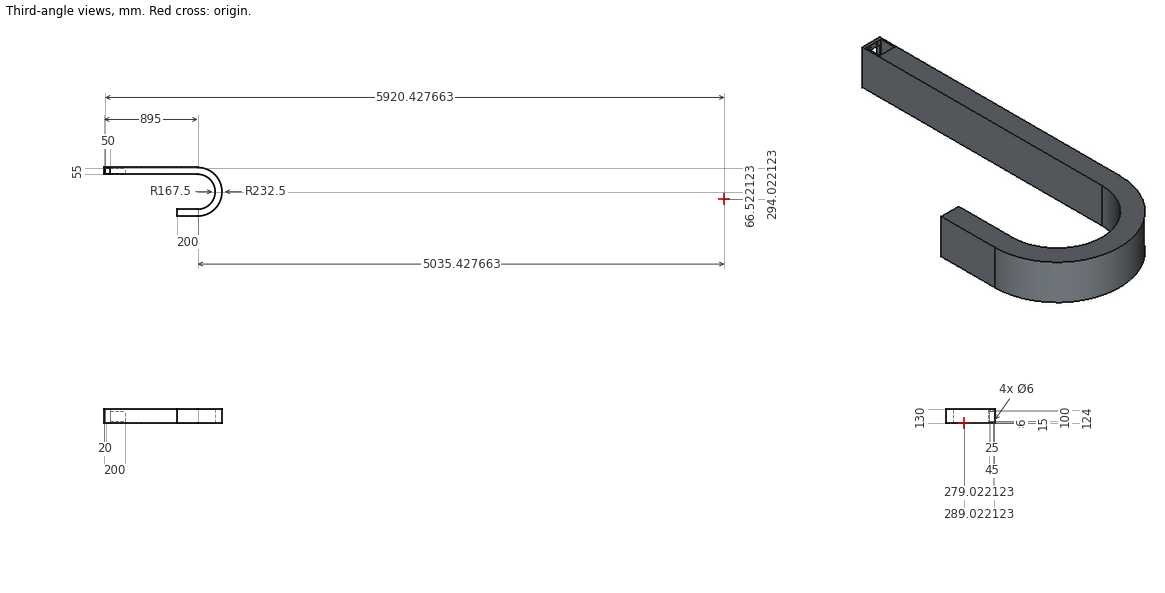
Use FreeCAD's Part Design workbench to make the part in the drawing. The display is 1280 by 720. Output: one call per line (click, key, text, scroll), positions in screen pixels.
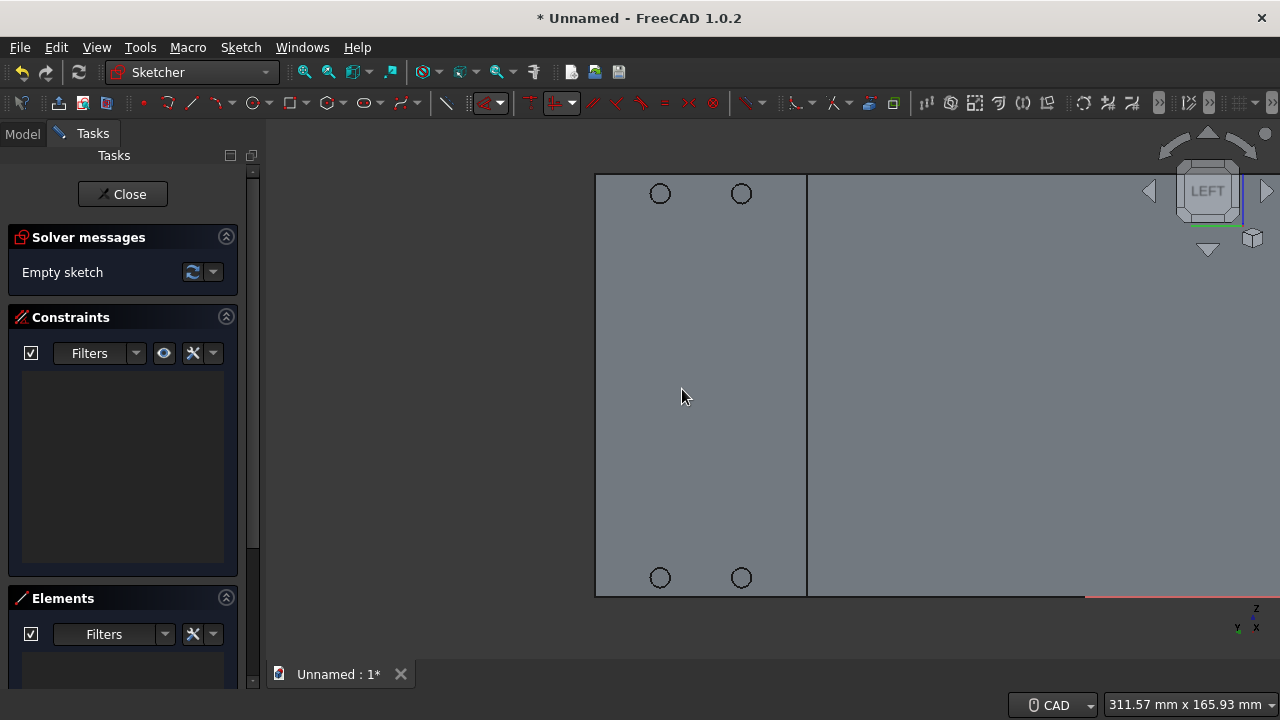
click(290, 104)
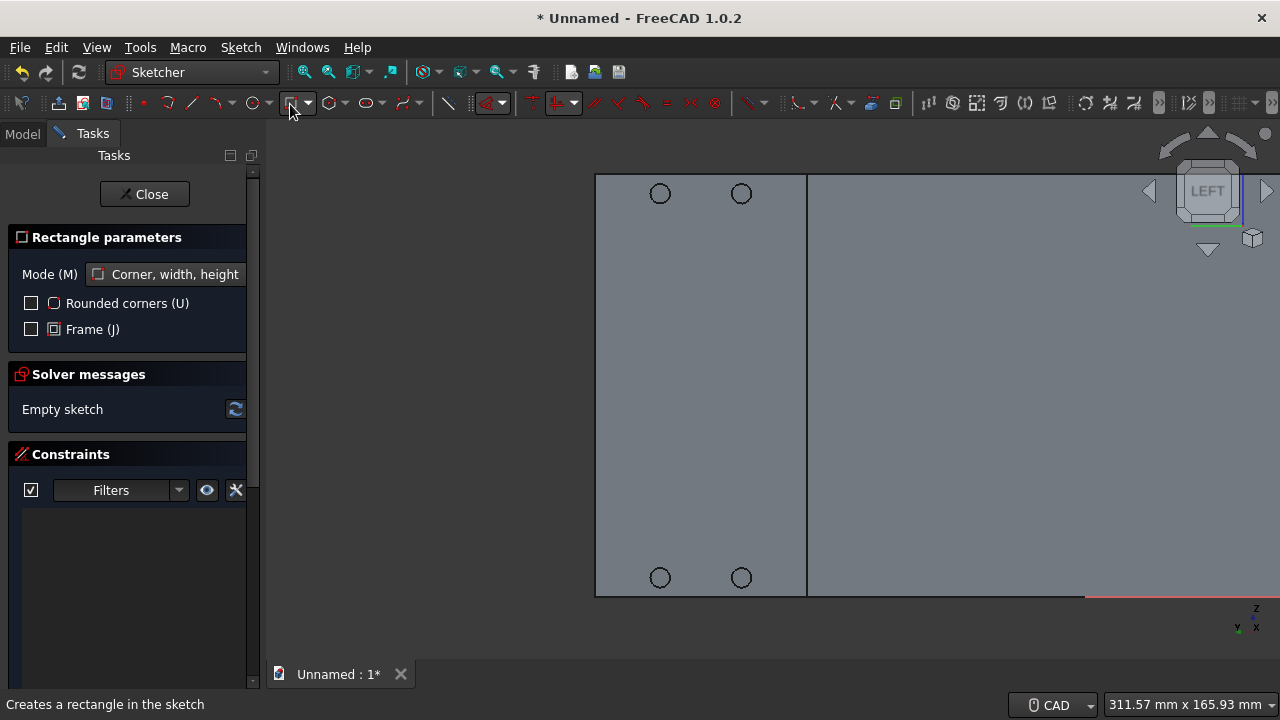
click(628, 223)
move(774, 549)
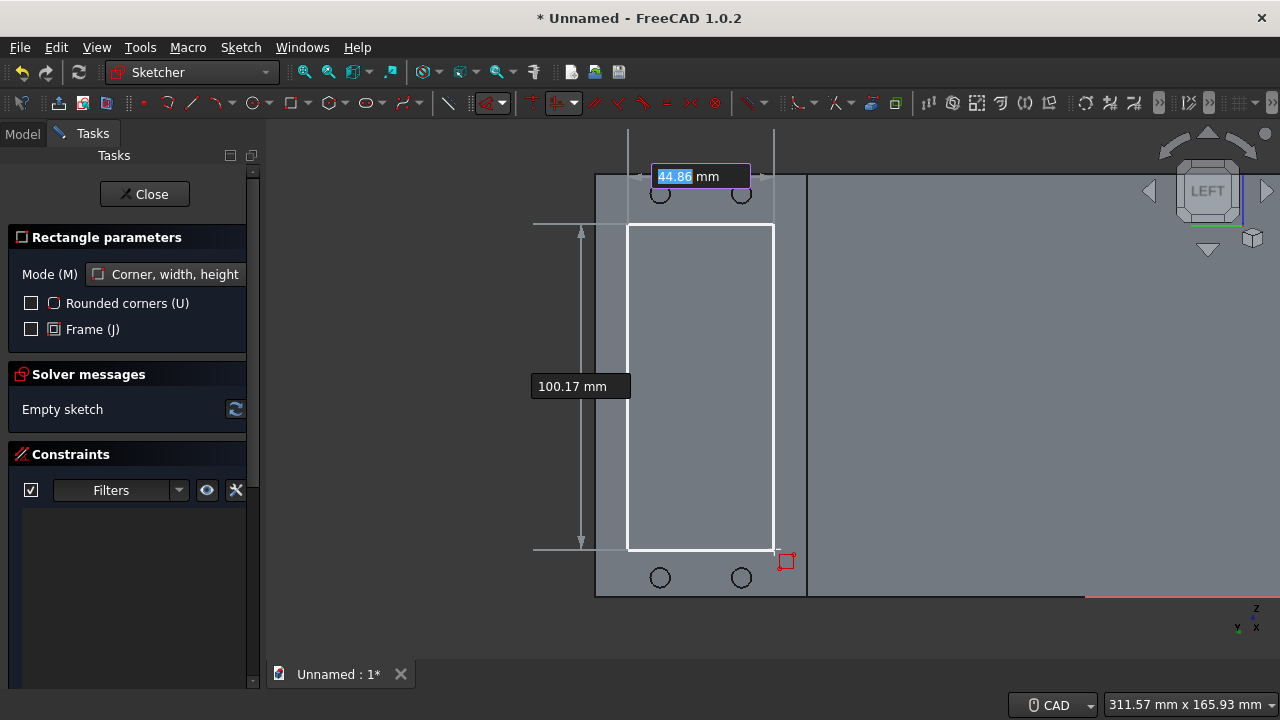
text(45)
key(Tab)
text(100)
key(Return)
key(Escape)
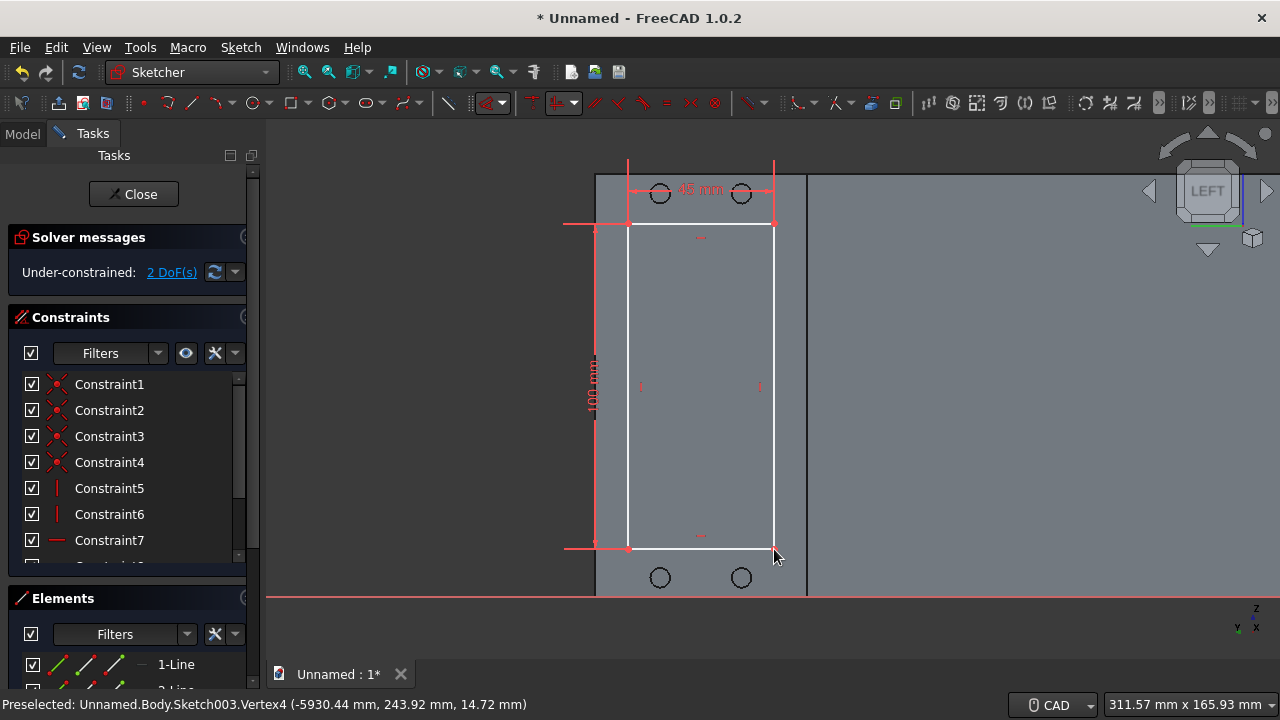
click(628, 549)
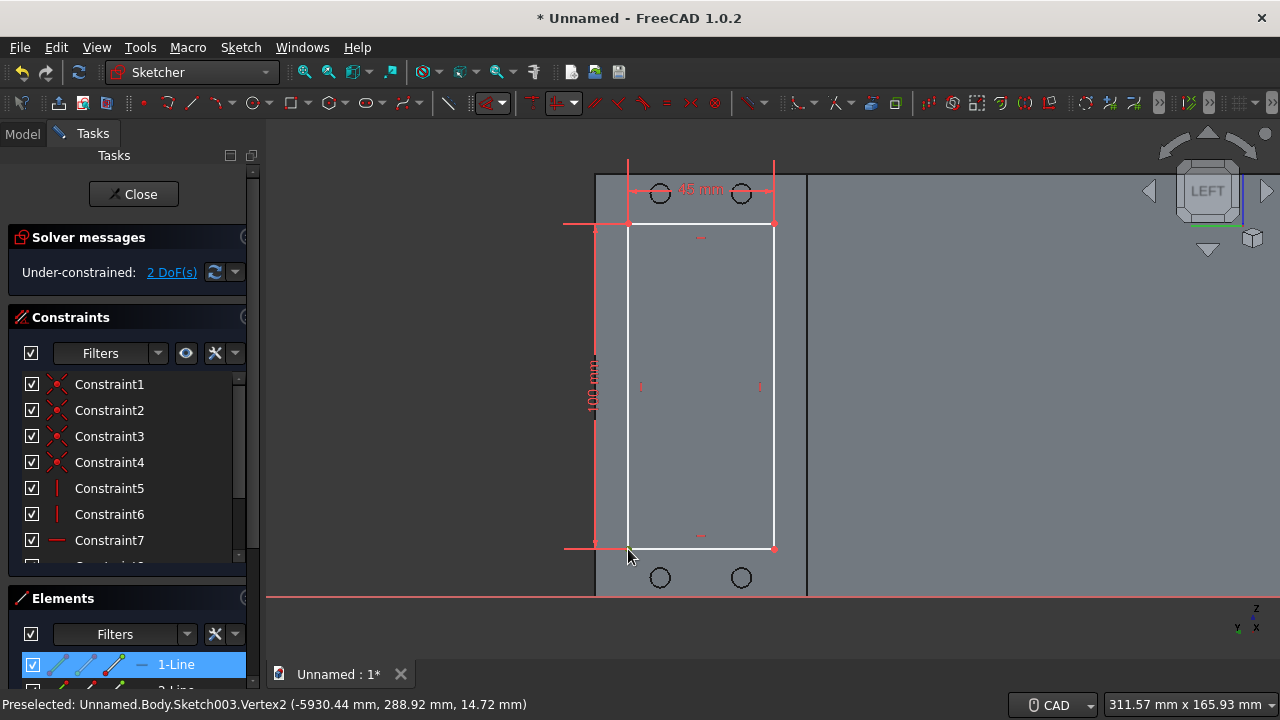
key(i)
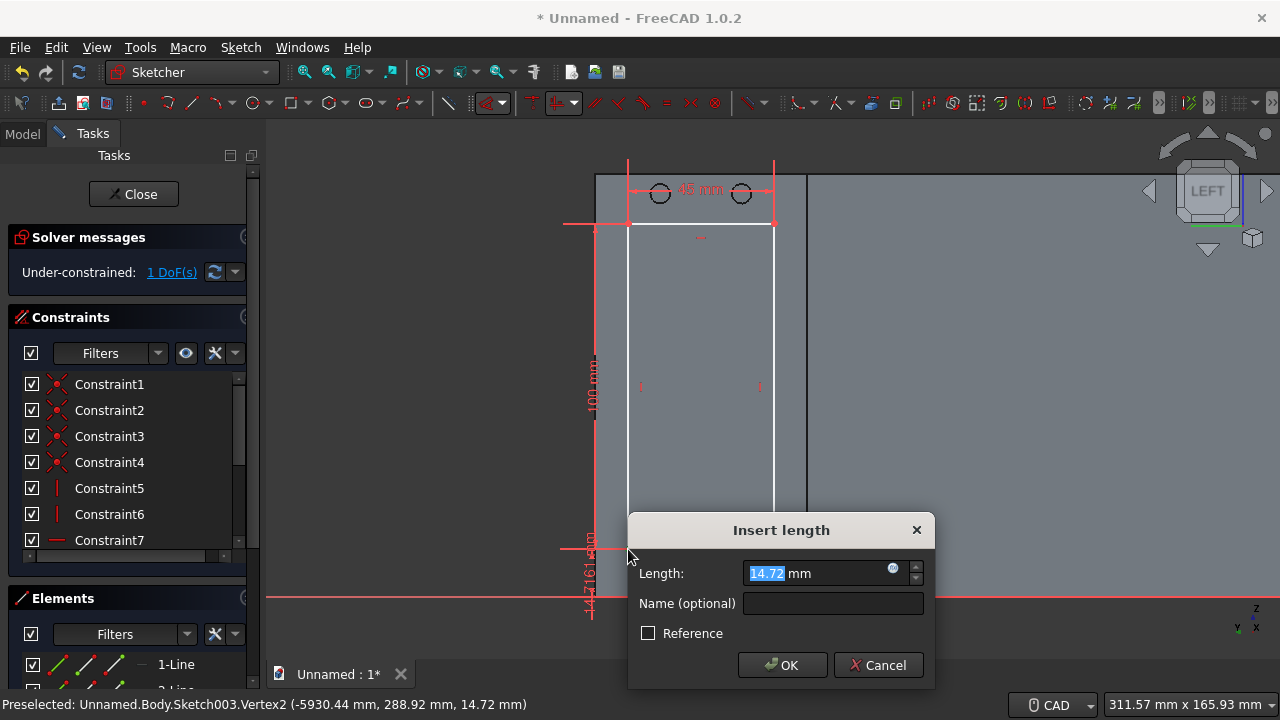
text(15)
key(Return)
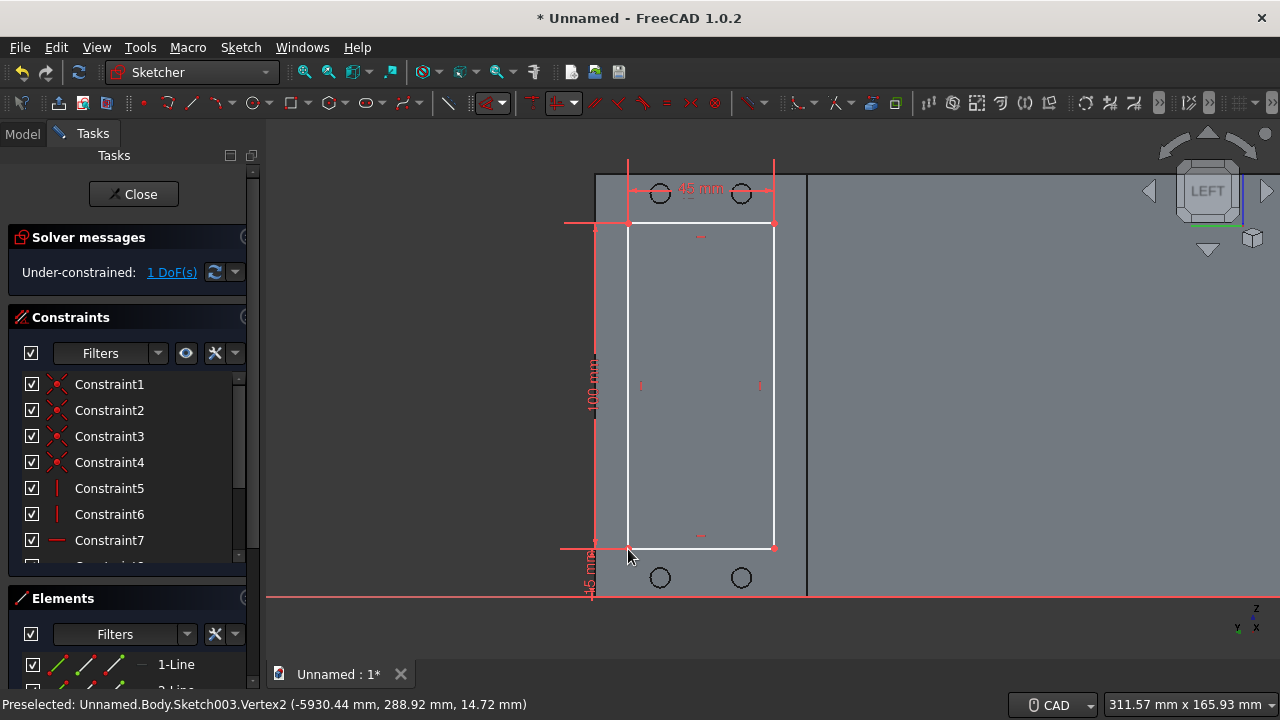
click(628, 223)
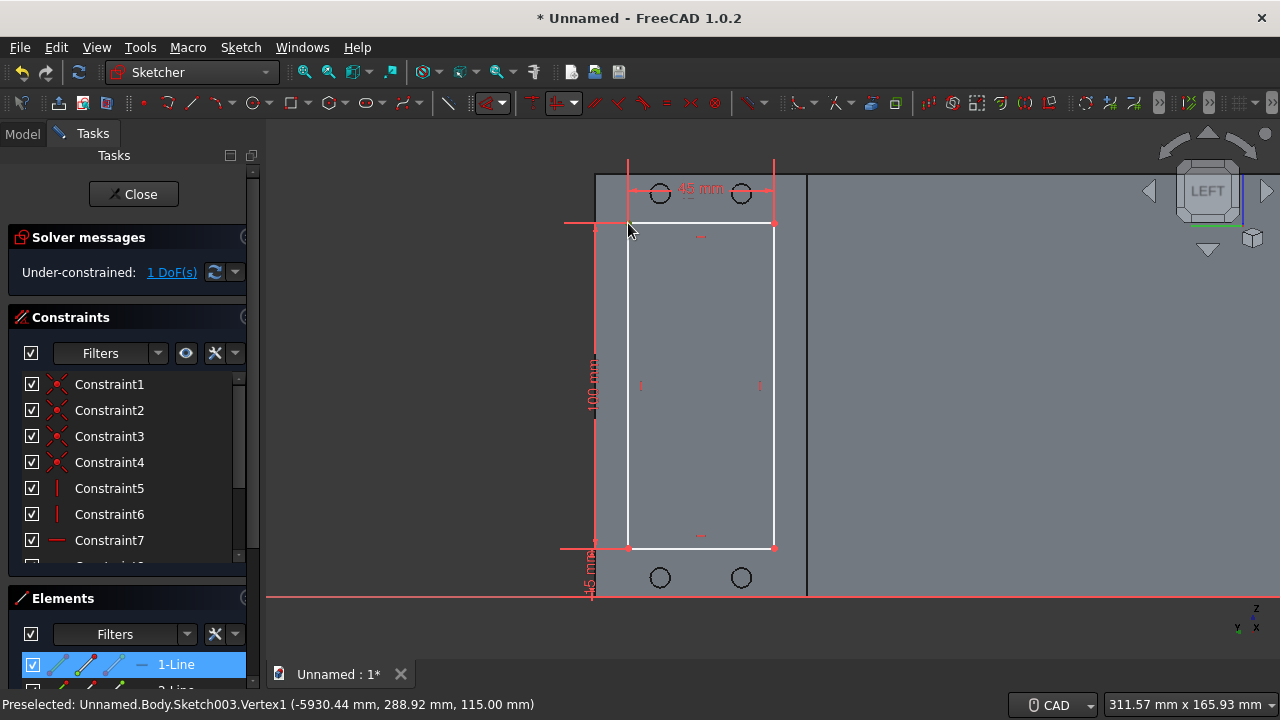
key(l)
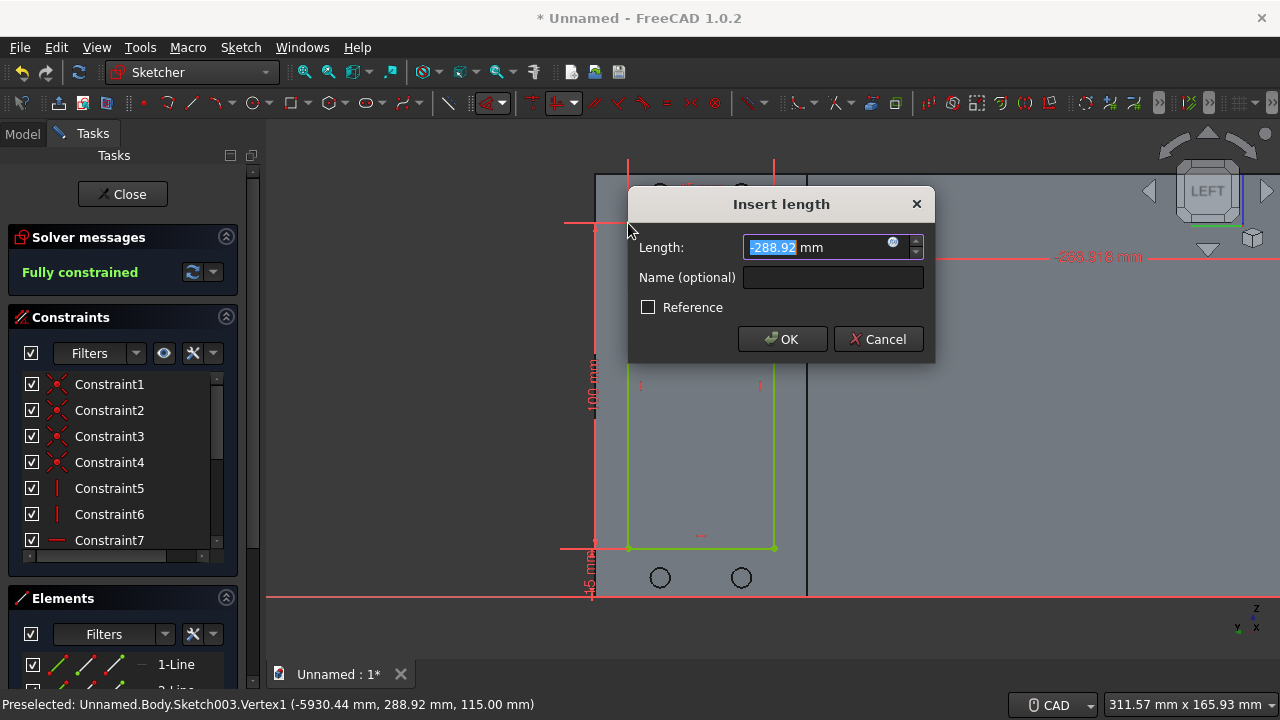
text(-289.022123)
key(Return)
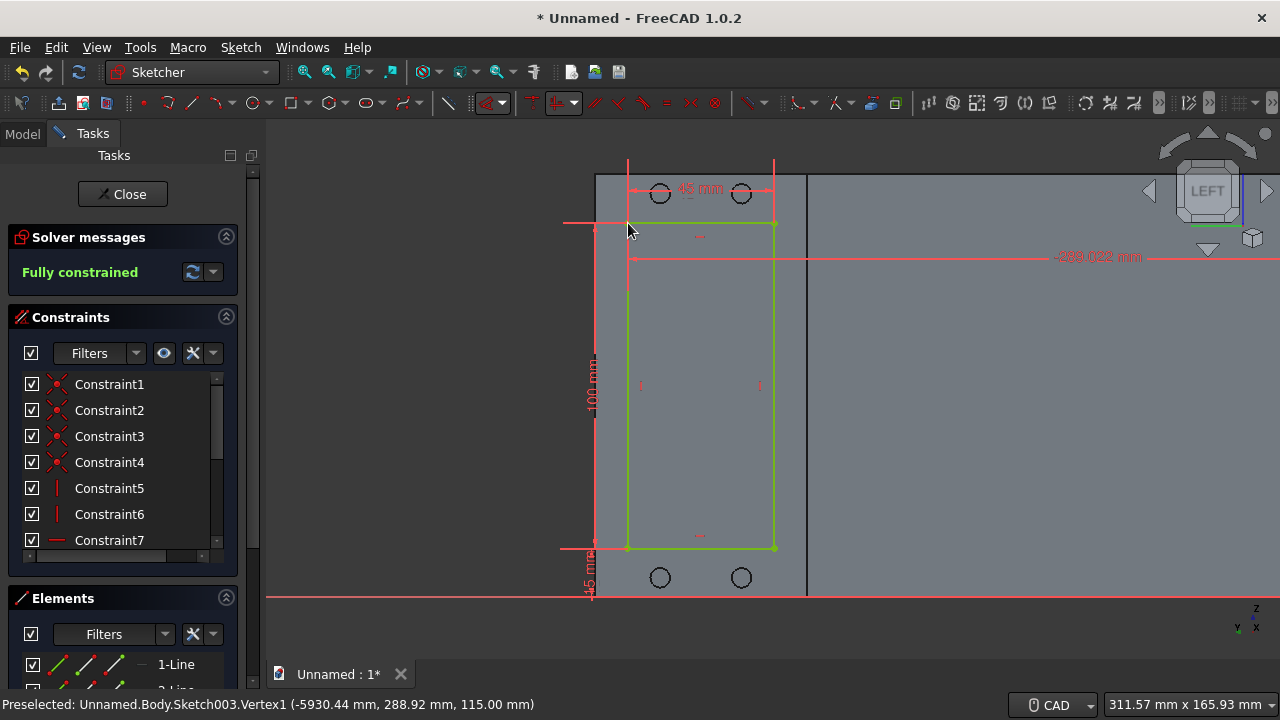
click(123, 194)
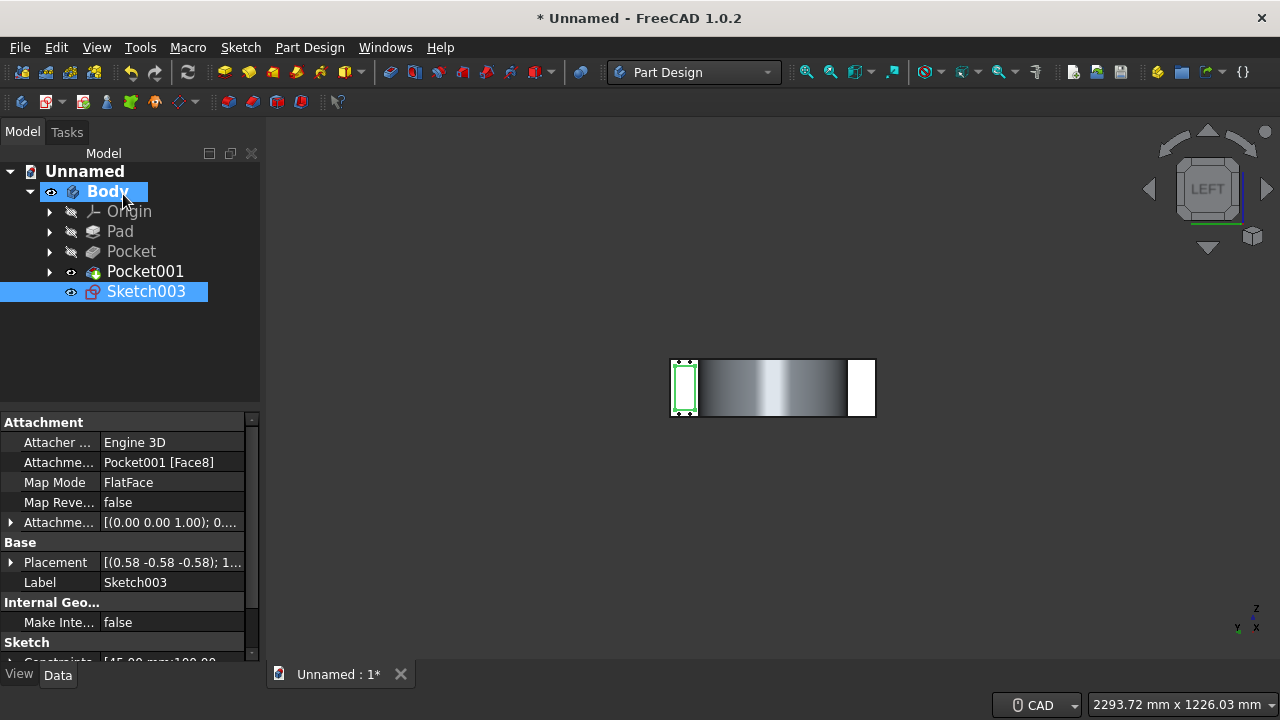
click(392, 72)